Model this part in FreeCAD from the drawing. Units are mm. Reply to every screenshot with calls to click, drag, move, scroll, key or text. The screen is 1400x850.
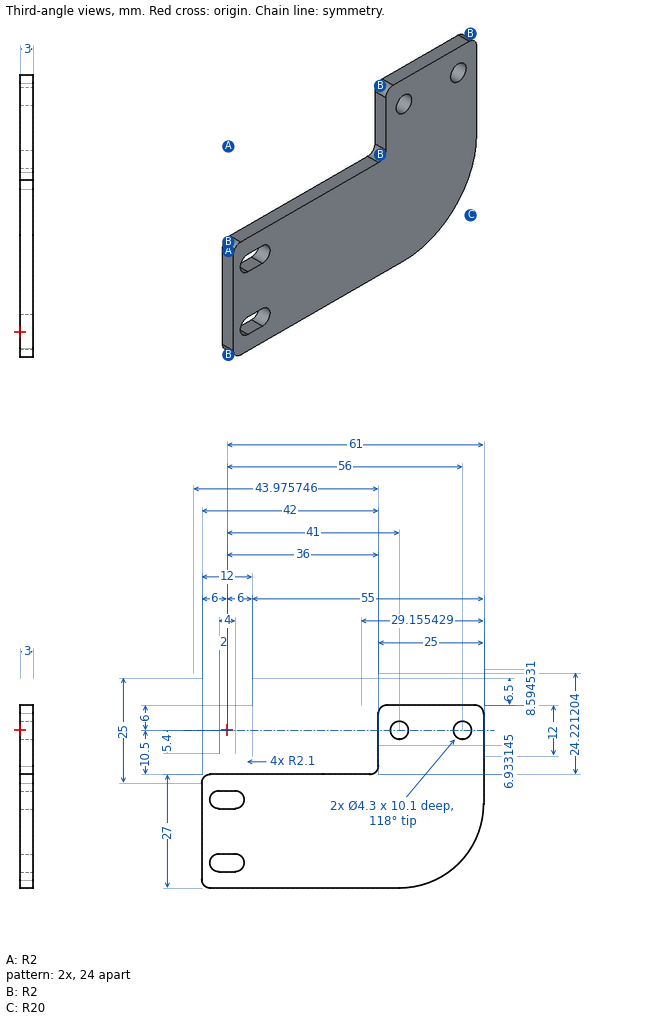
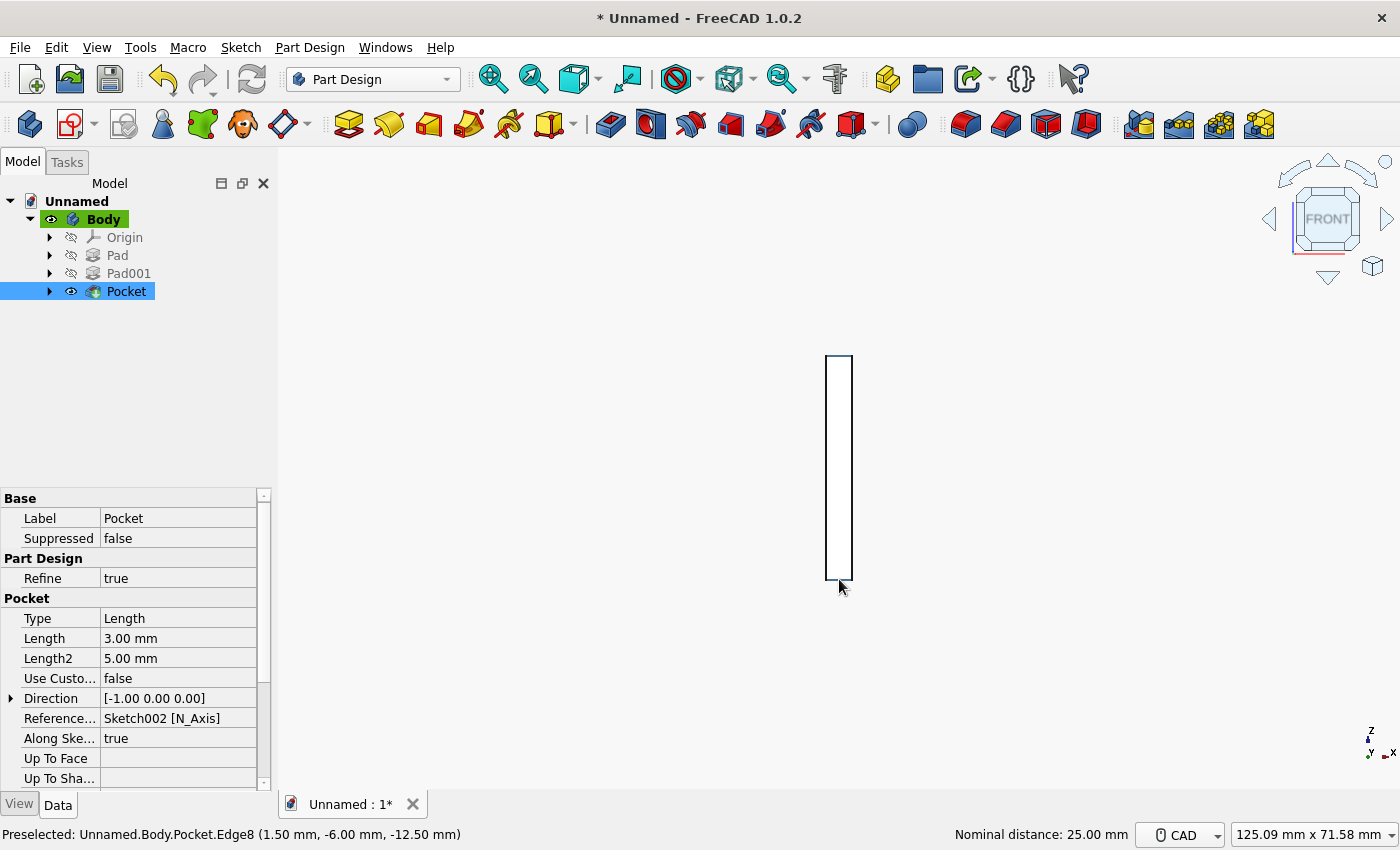
click(966, 124)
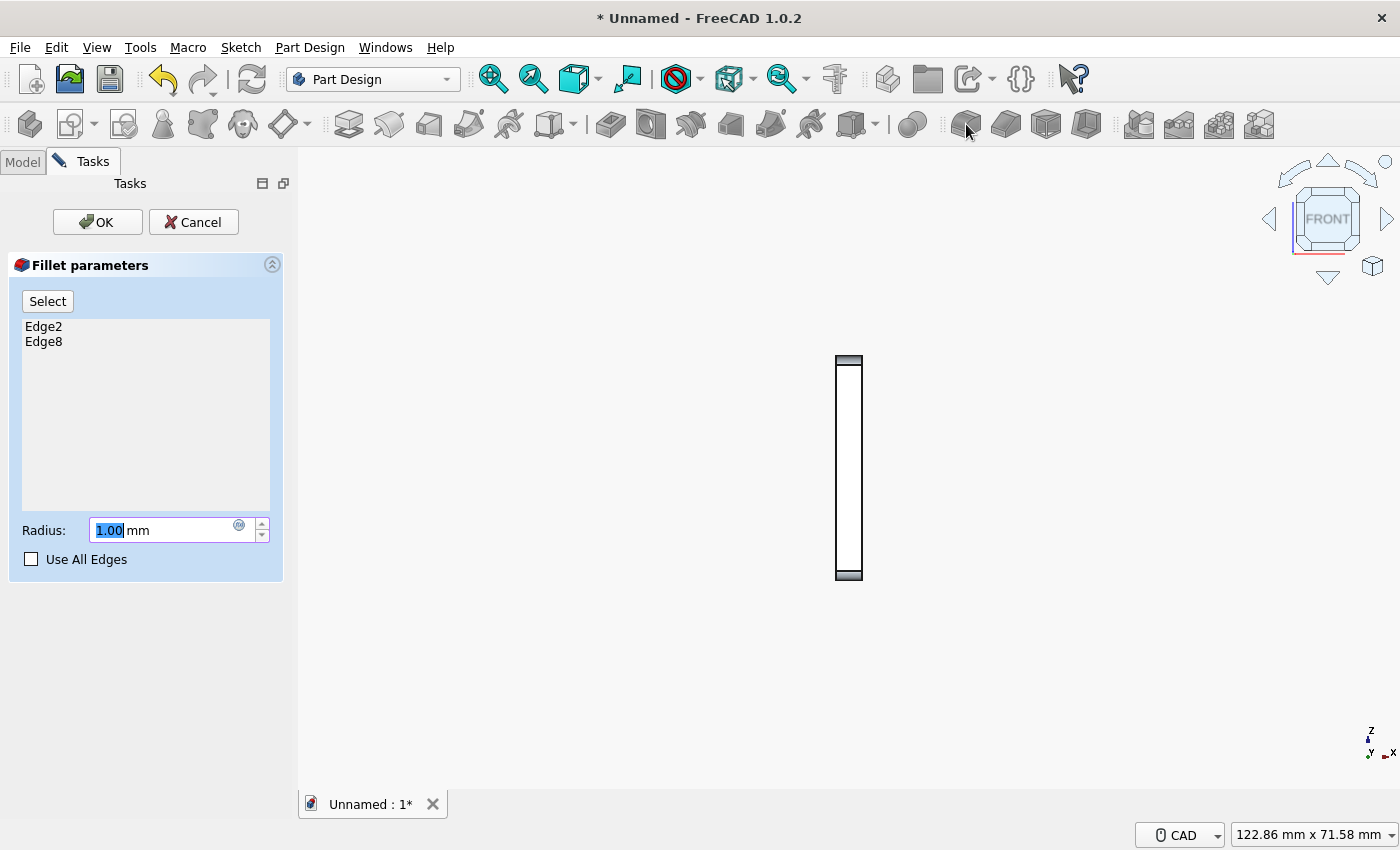
text(2)
key(Tab)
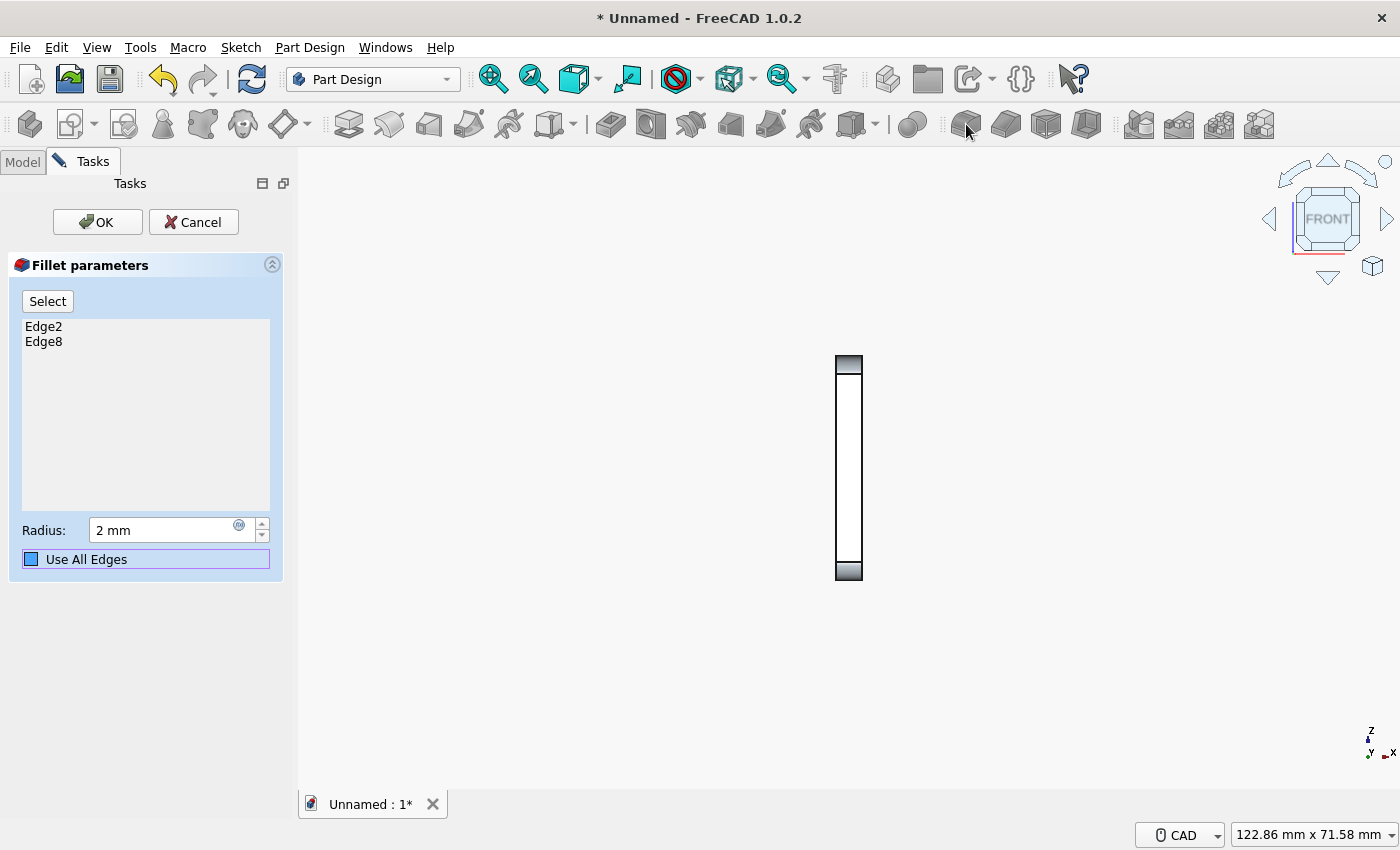
click(98, 222)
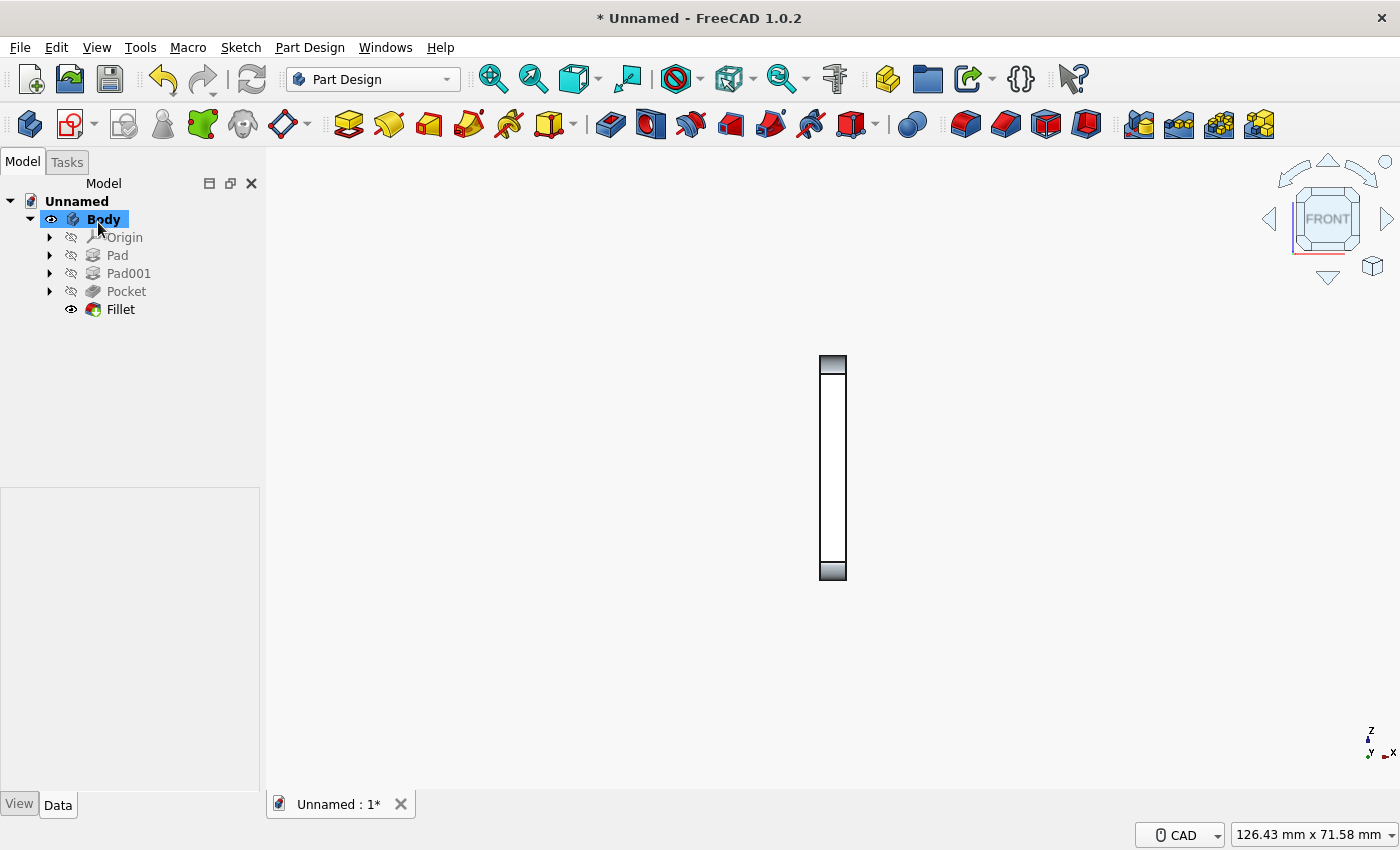
click(494, 80)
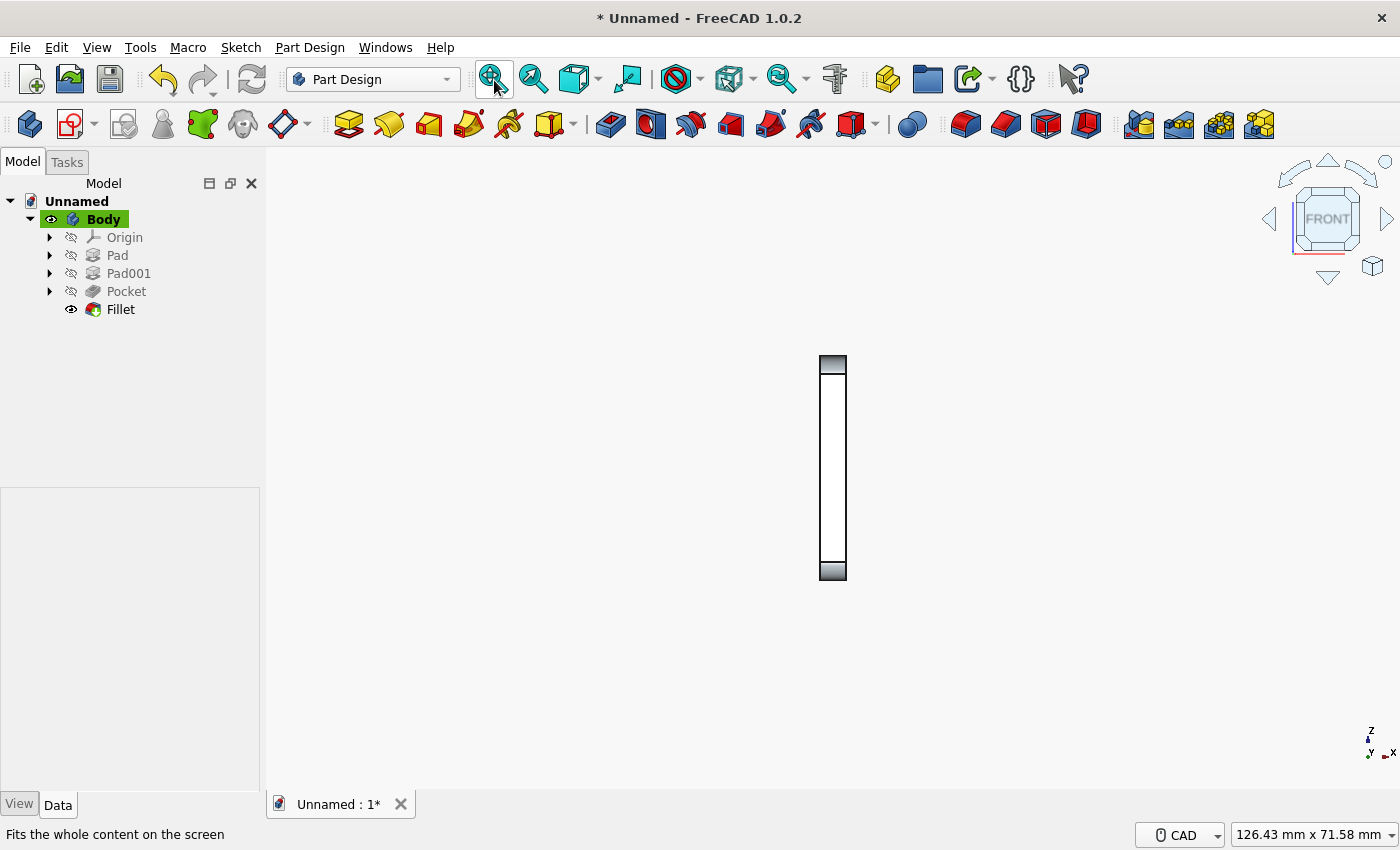
key(6)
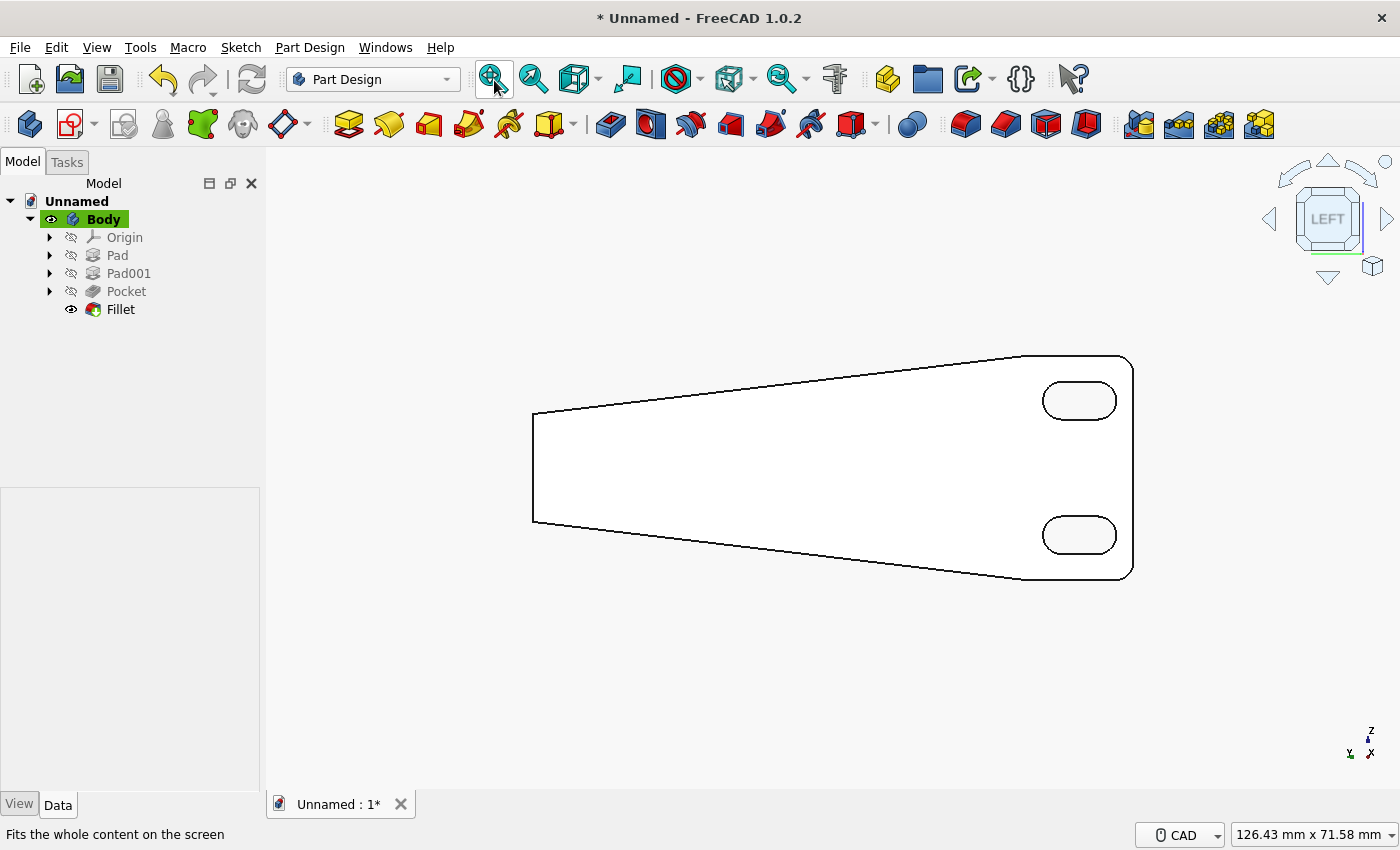
click(919, 467)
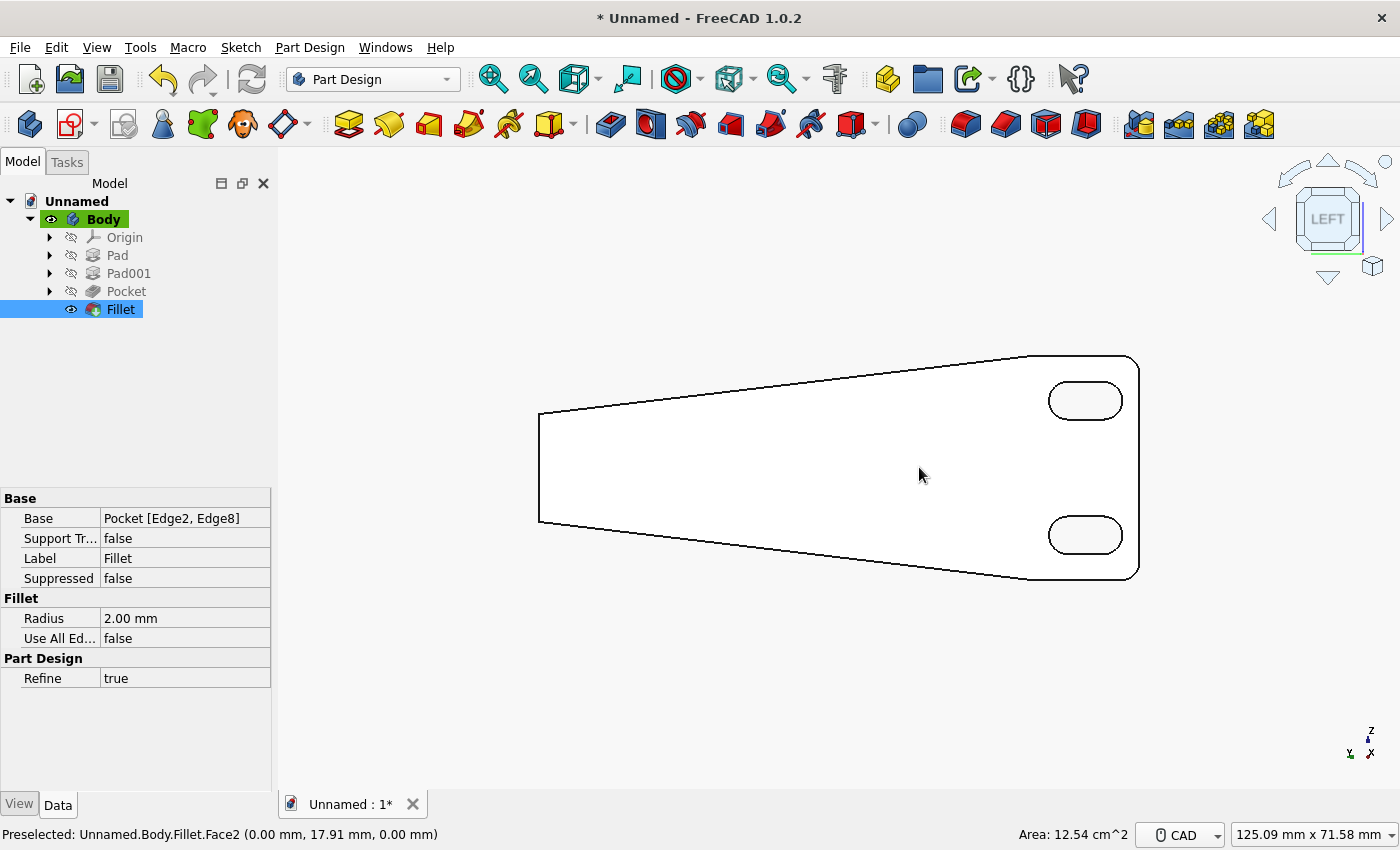
click(70, 124)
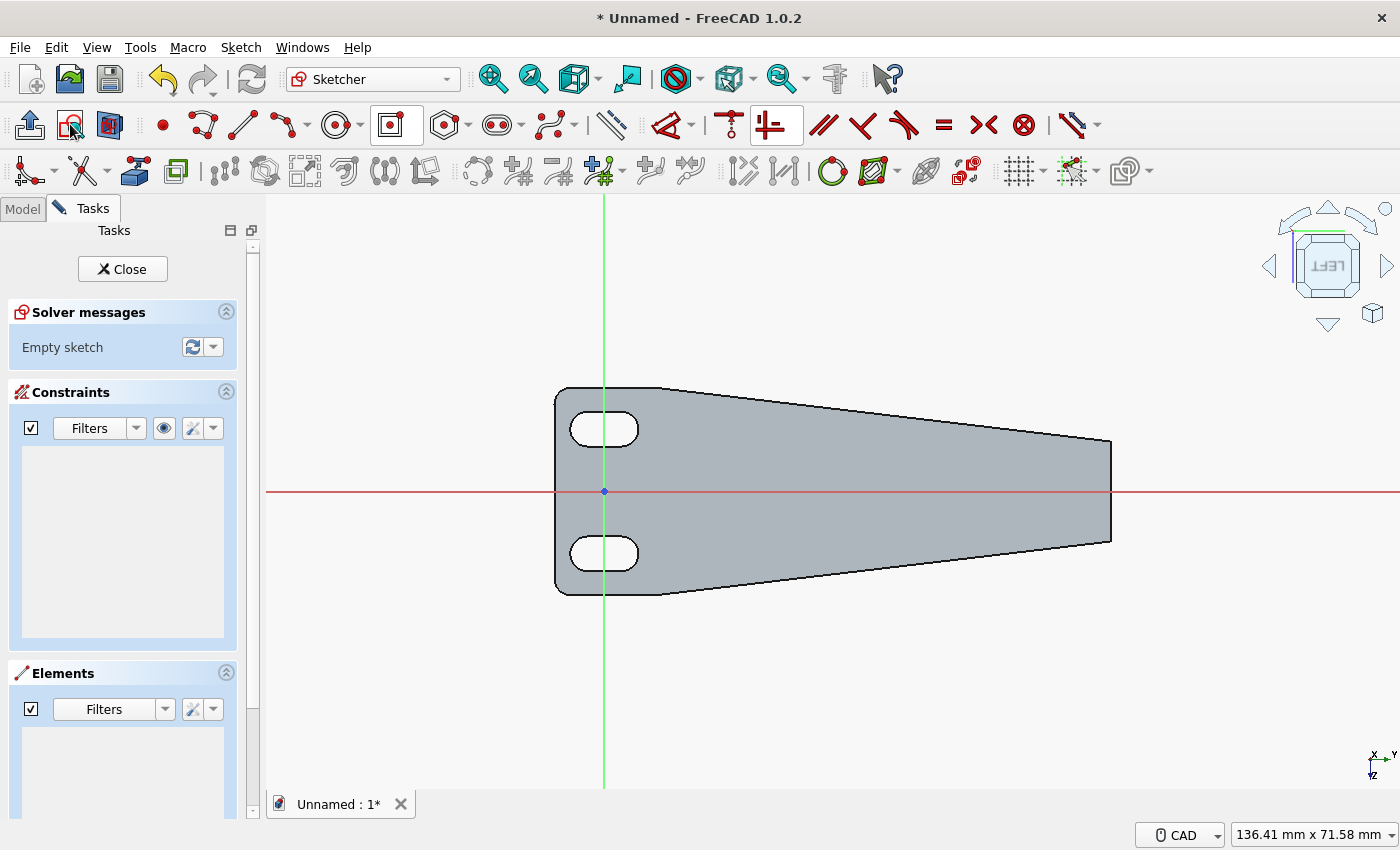
scroll(1087, 492, up, 7)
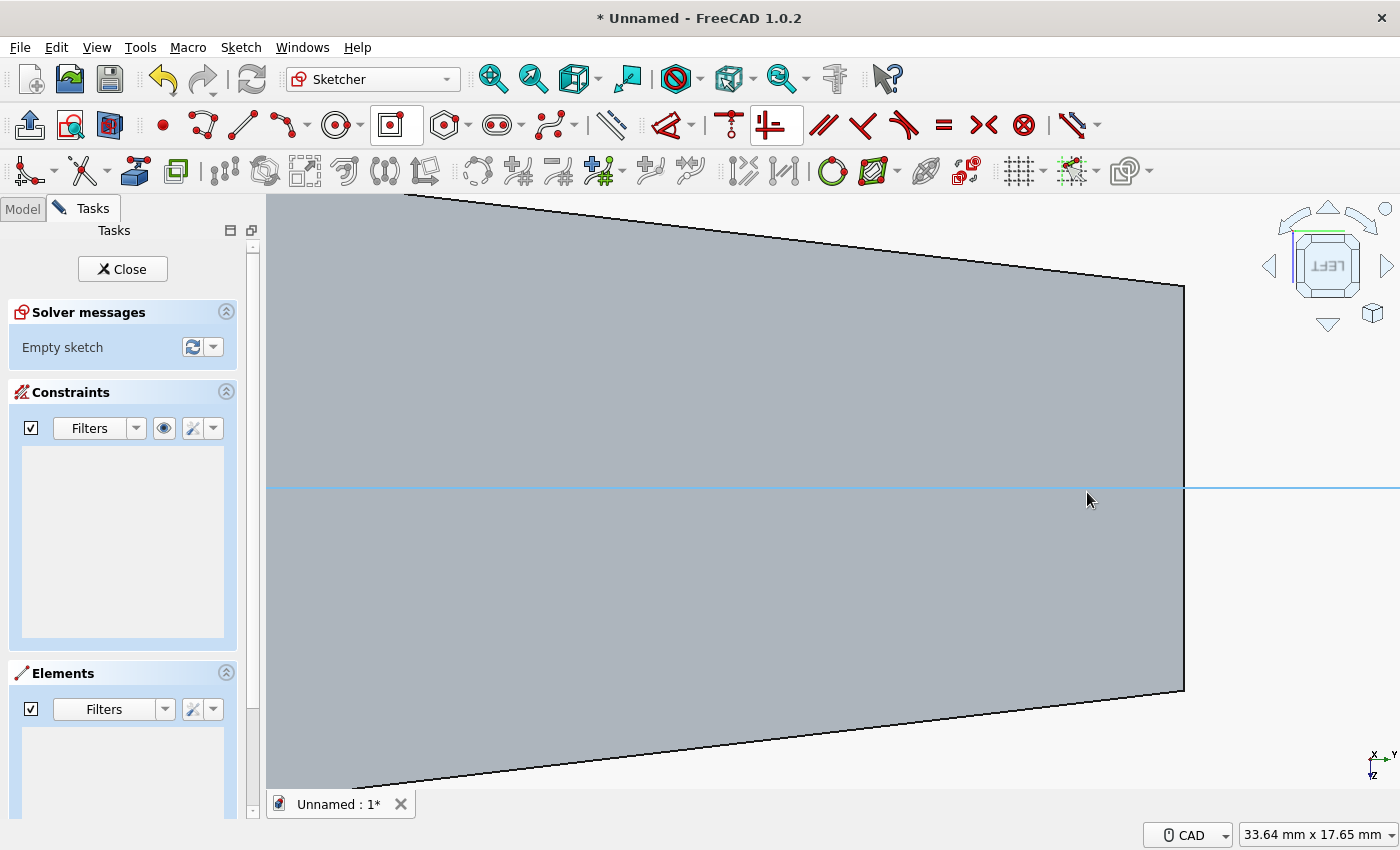
click(336, 126)